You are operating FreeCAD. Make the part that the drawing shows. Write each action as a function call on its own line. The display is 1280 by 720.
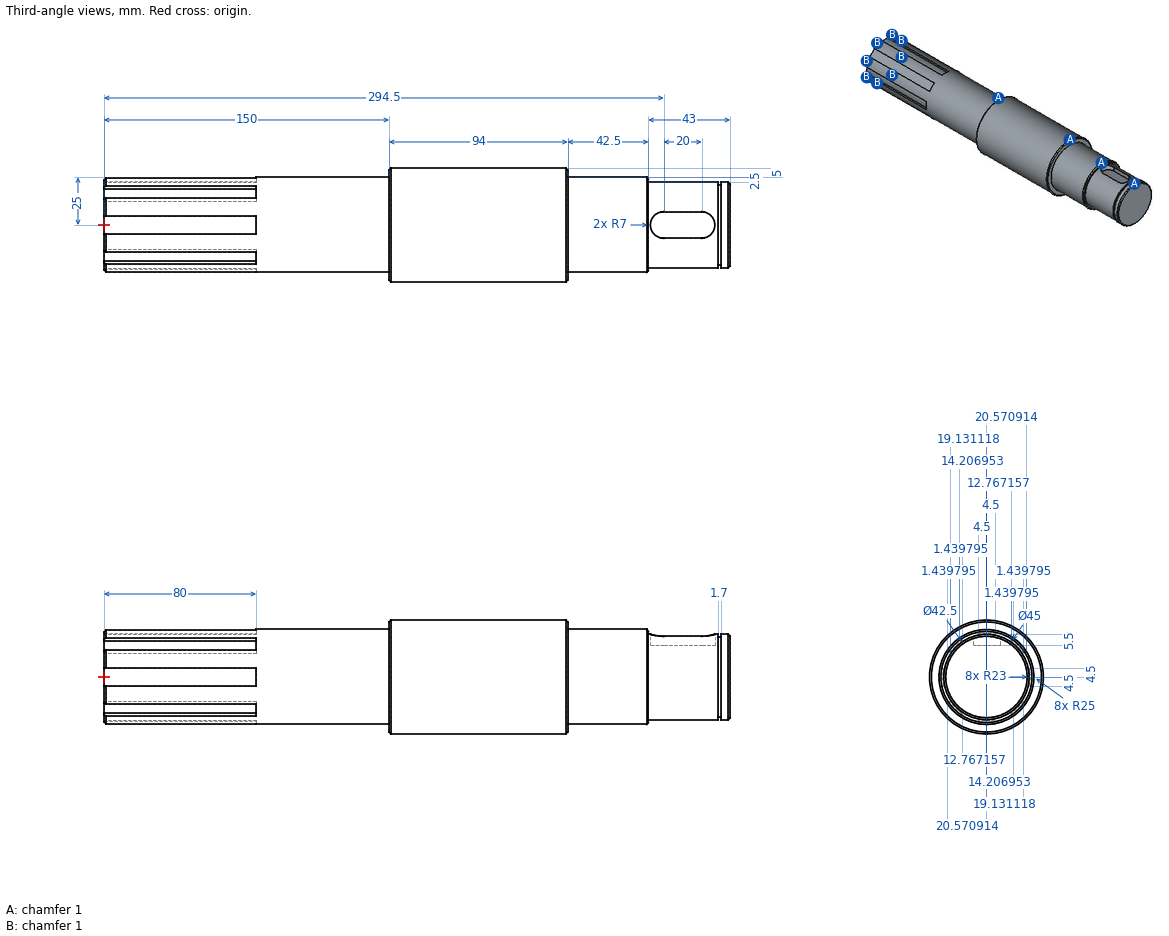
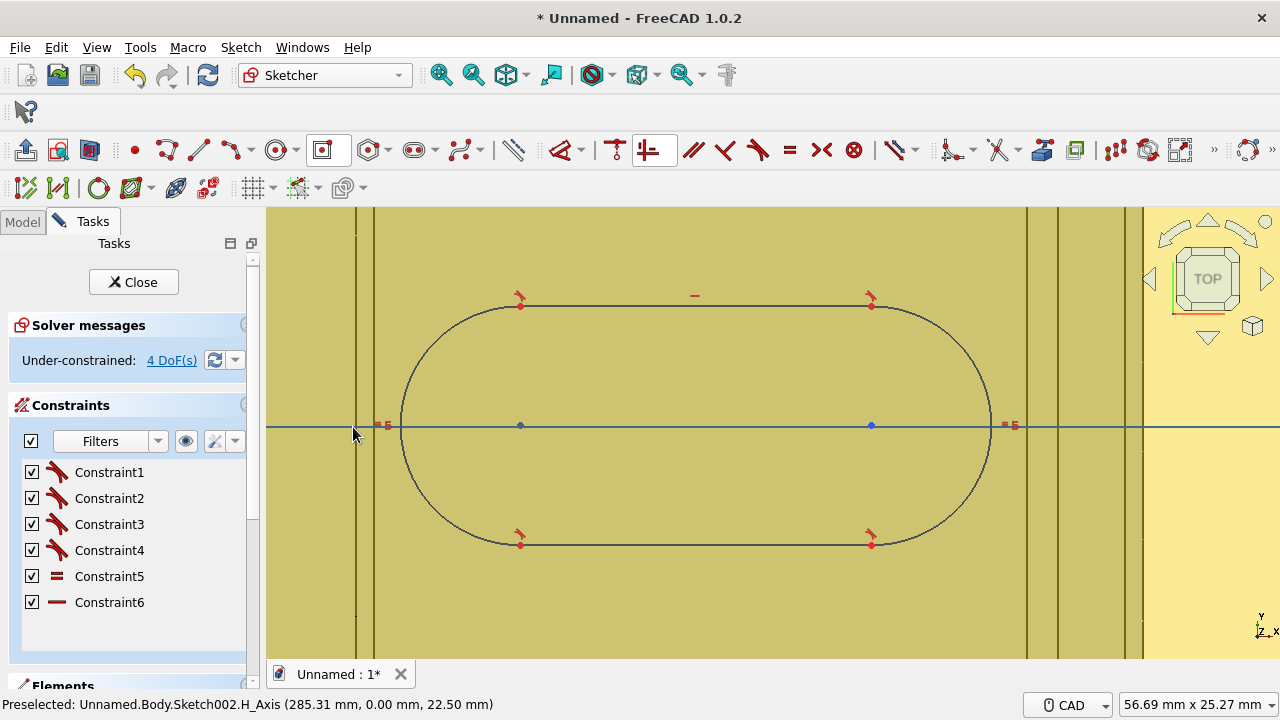
click(616, 150)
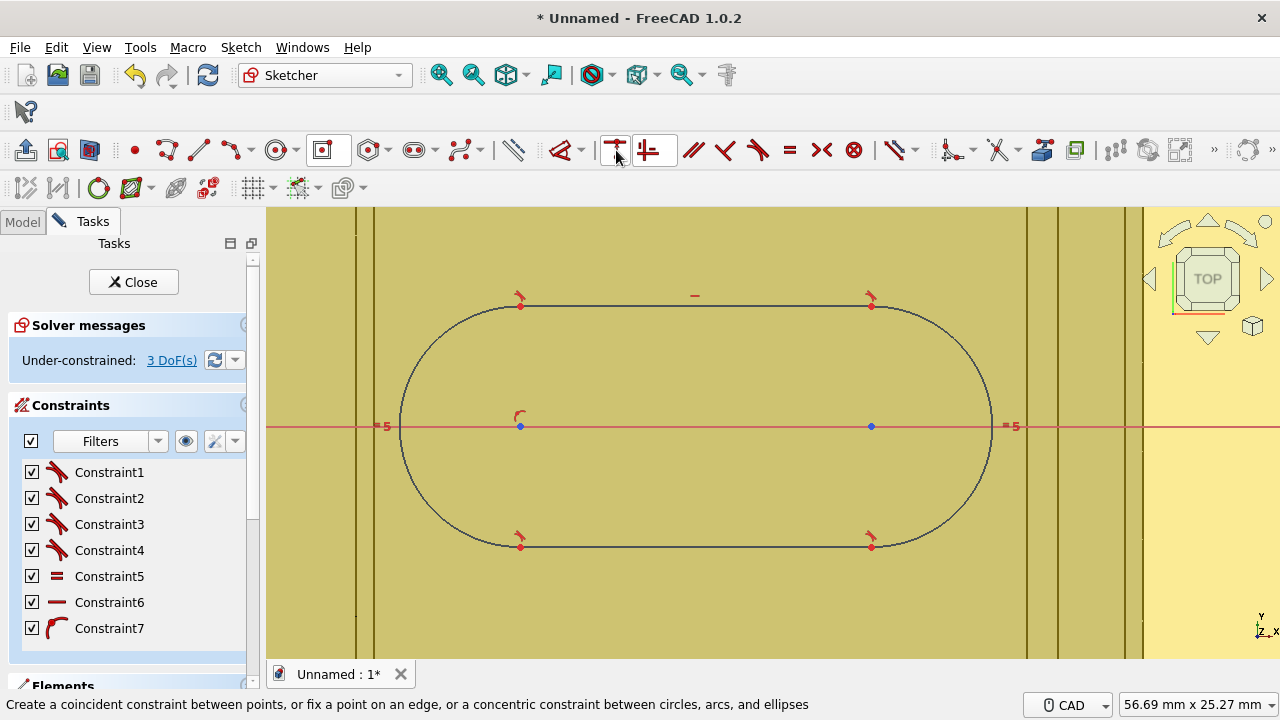
click(560, 150)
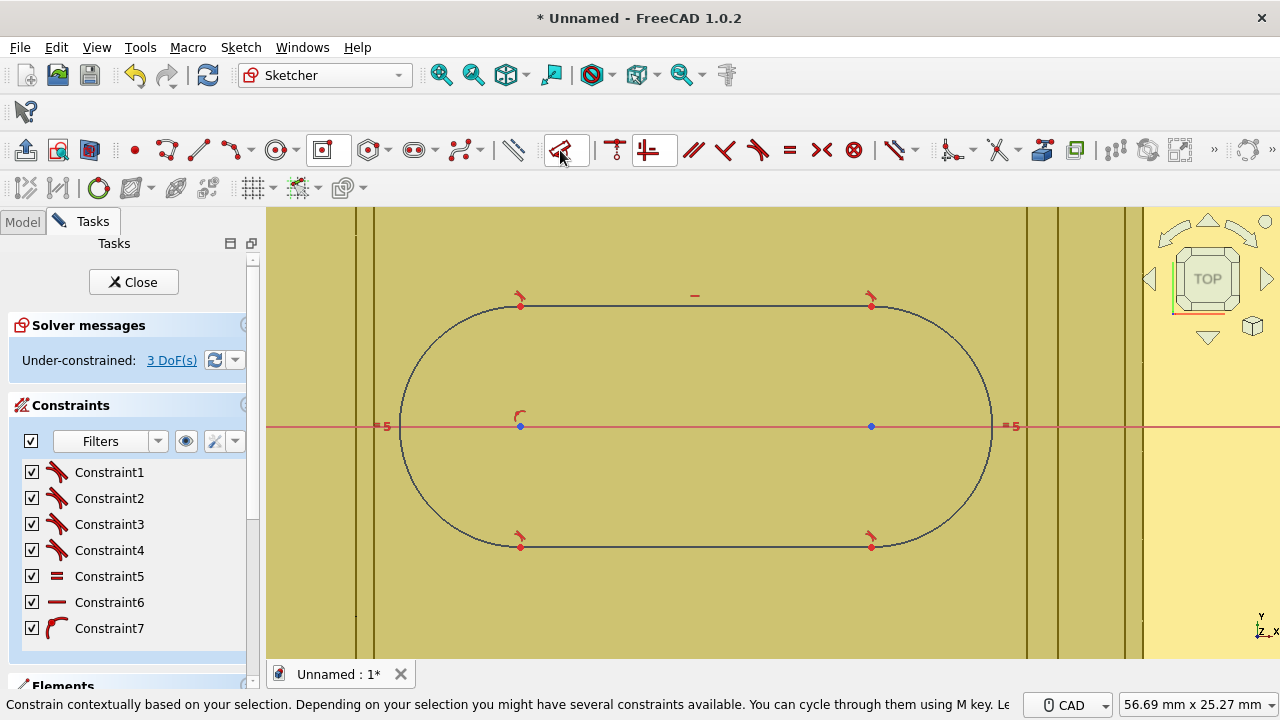
click(423, 356)
click(397, 337)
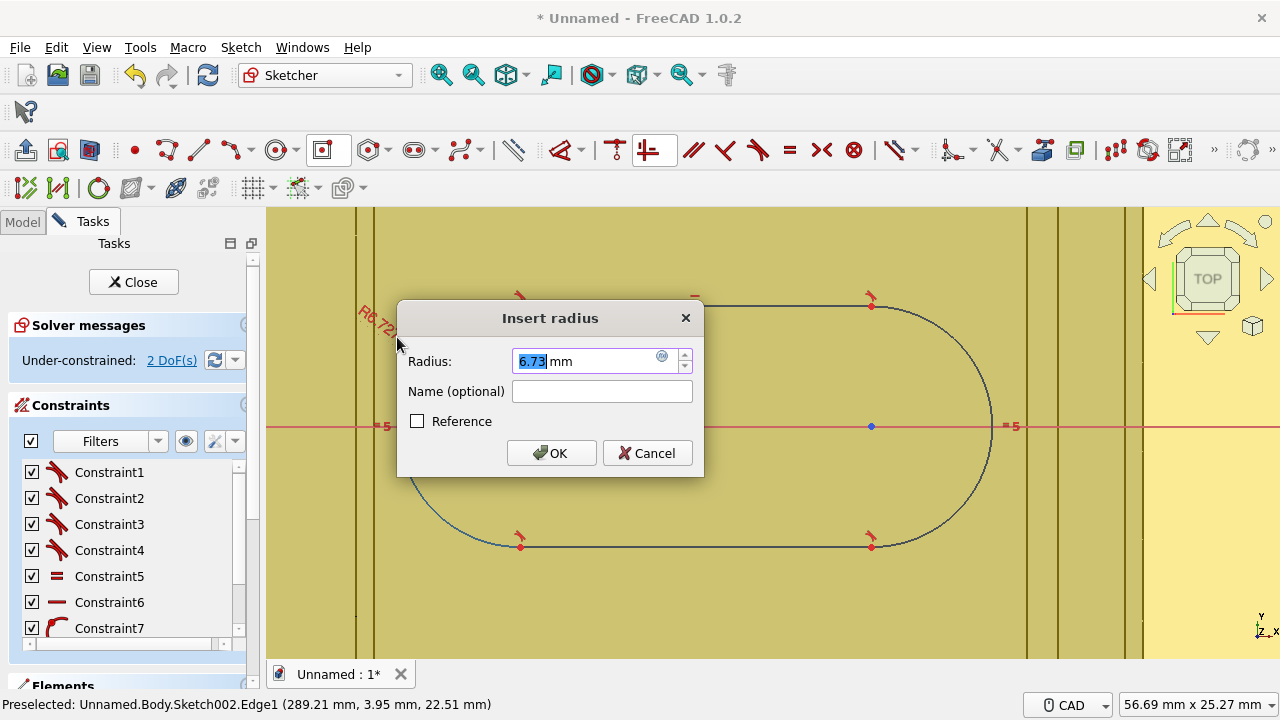
text(7)
key(Return)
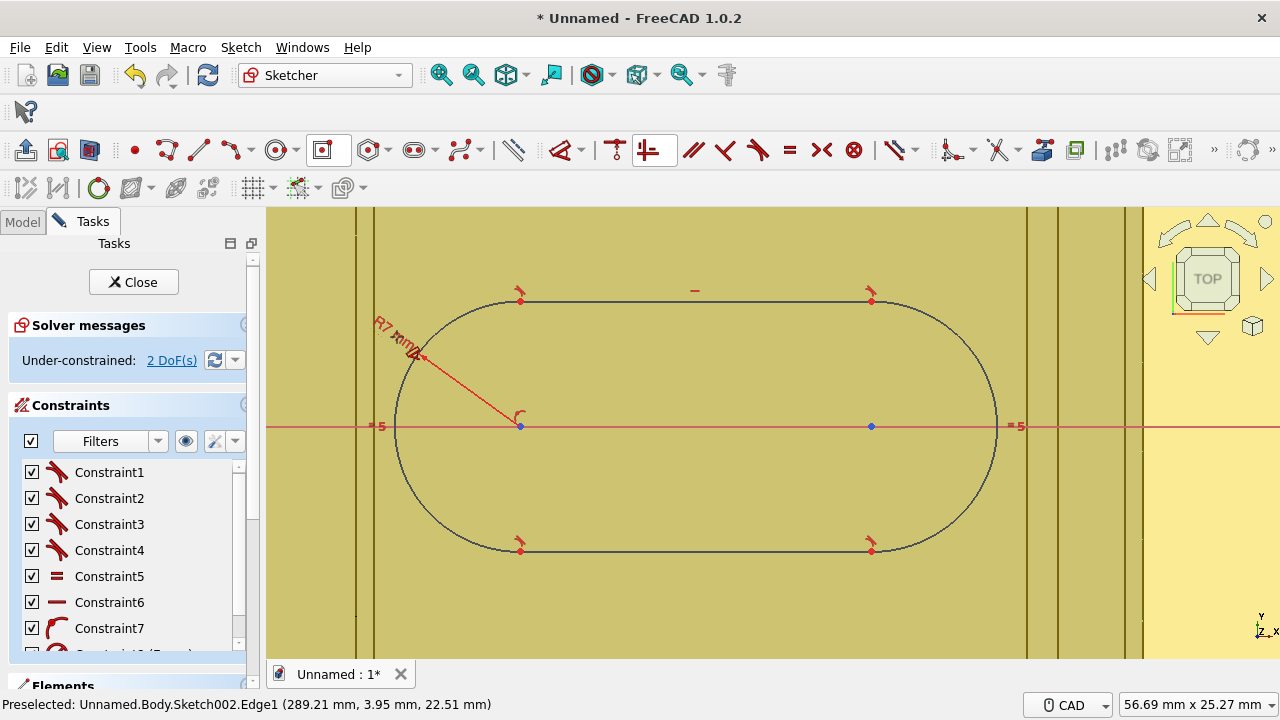
click(626, 302)
click(696, 268)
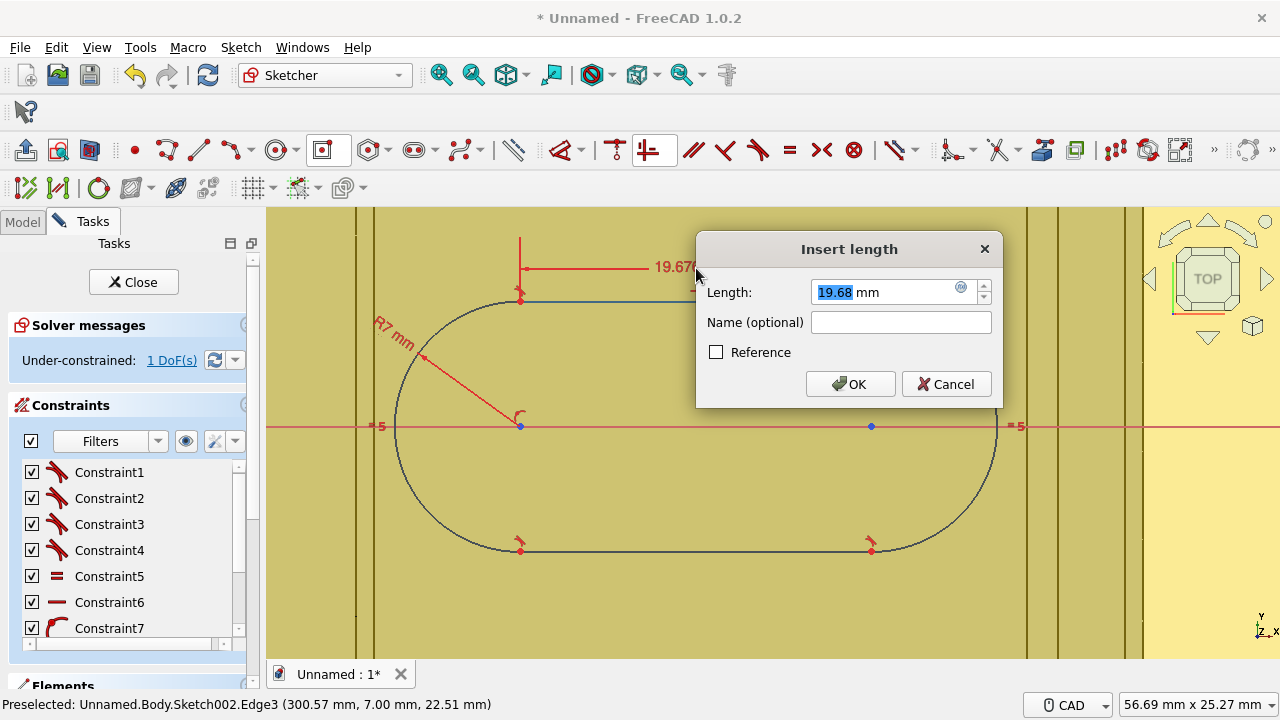
text(20)
key(Return)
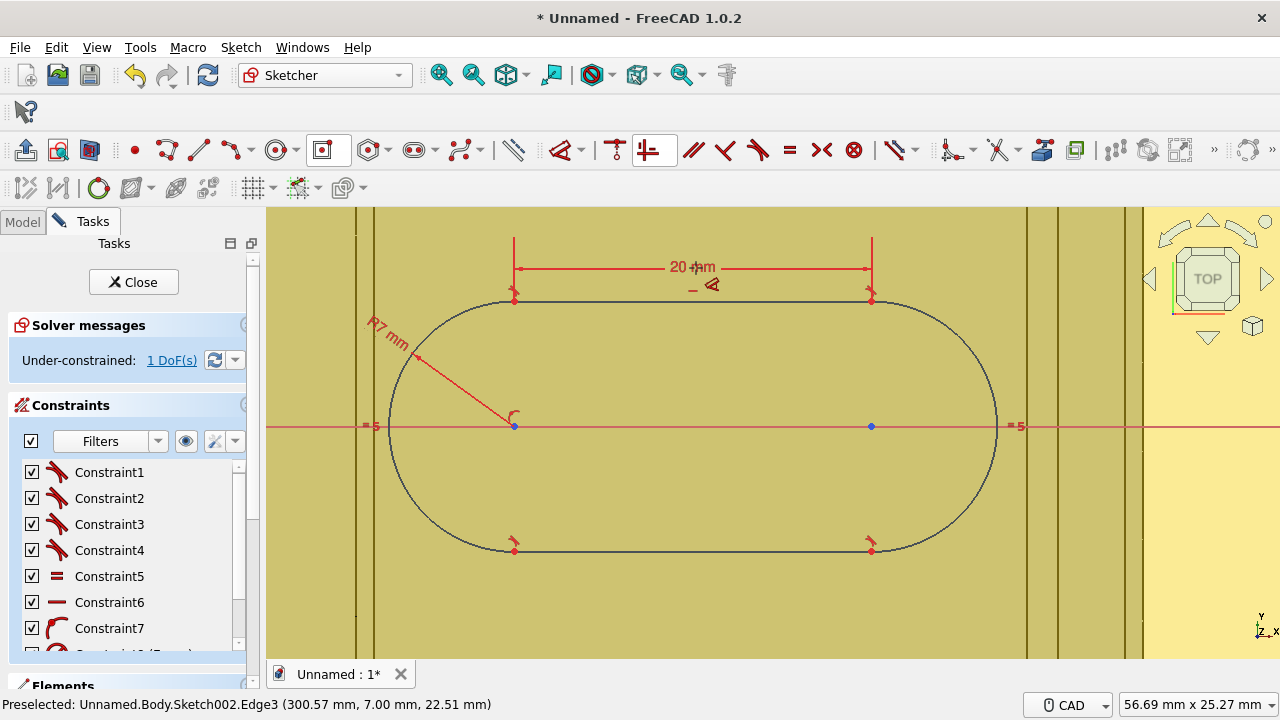
click(514, 302)
click(404, 268)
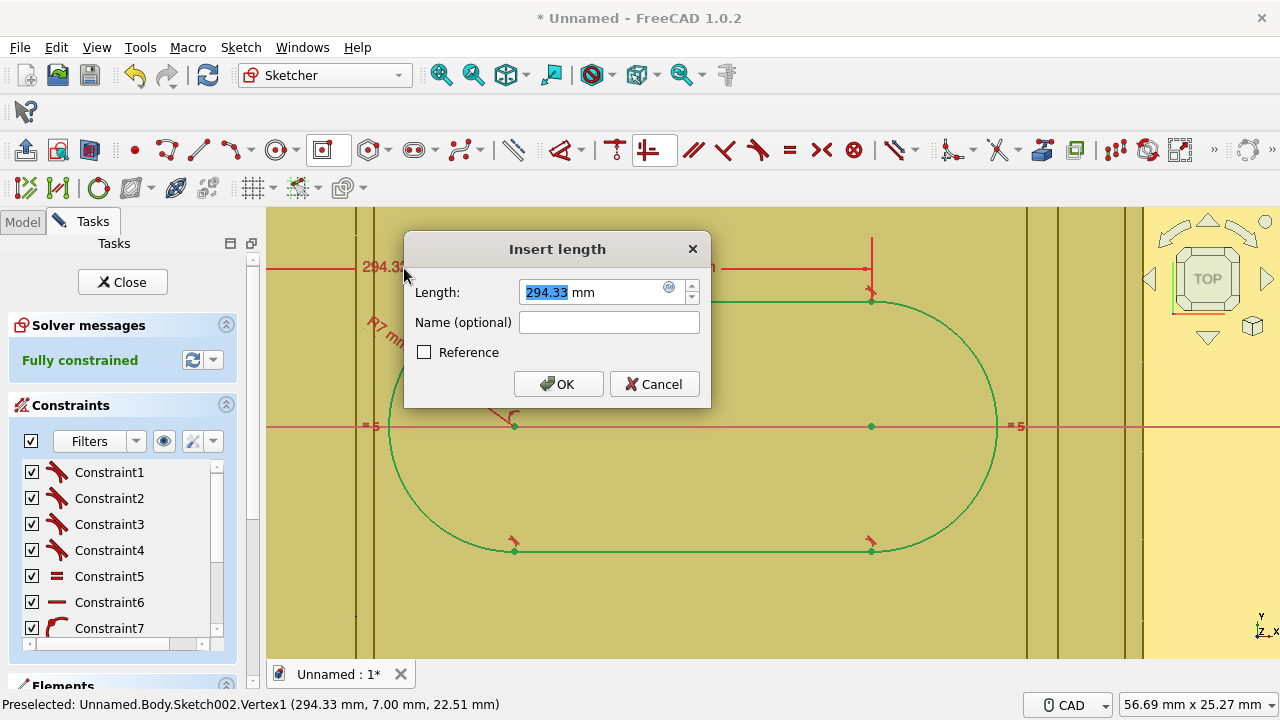
text(294.5)
key(Return)
key(Escape)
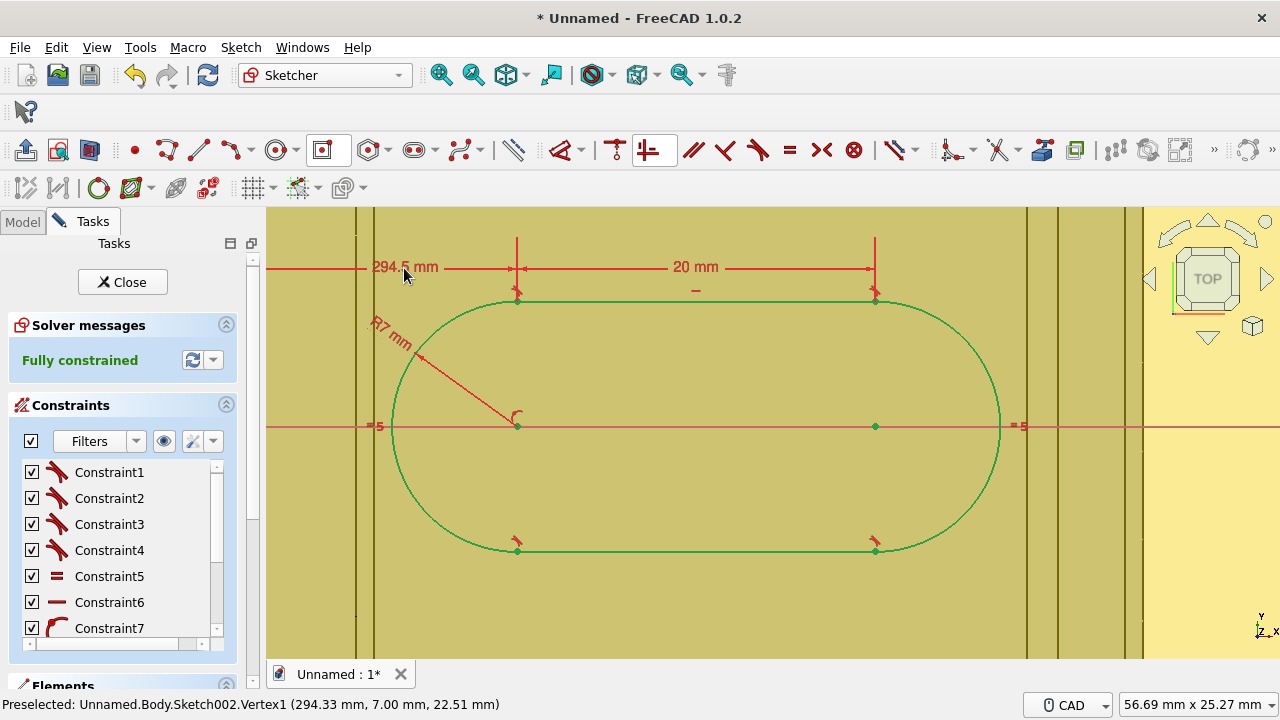
click(123, 282)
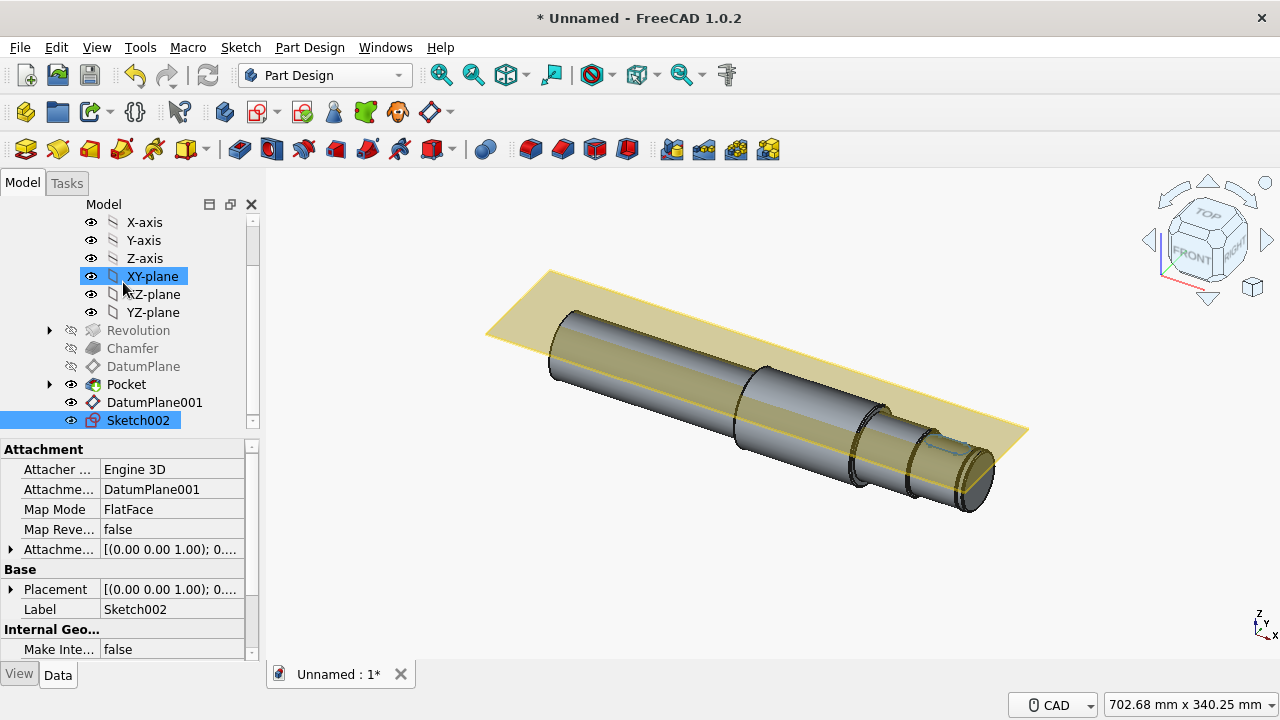
click(240, 150)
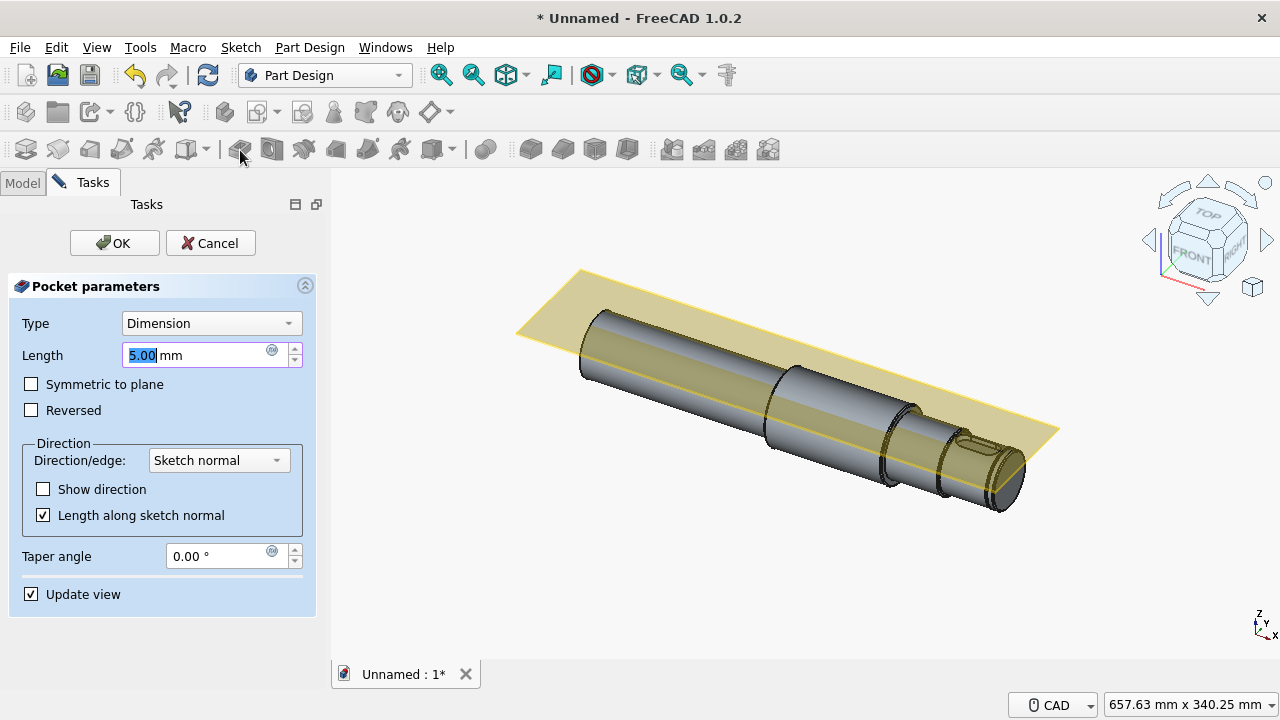
text(5.5)
key(Tab)